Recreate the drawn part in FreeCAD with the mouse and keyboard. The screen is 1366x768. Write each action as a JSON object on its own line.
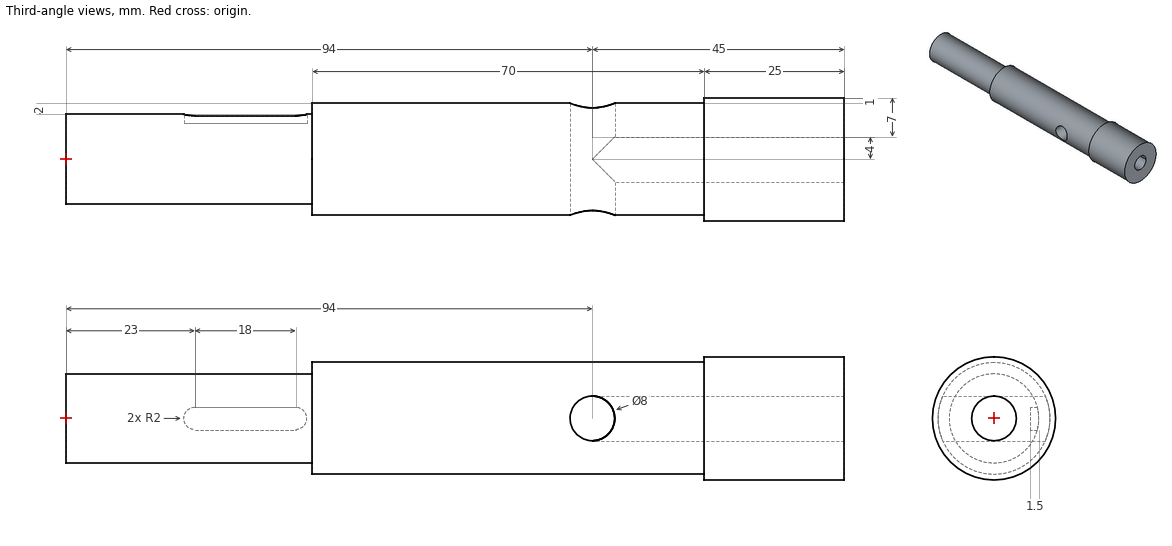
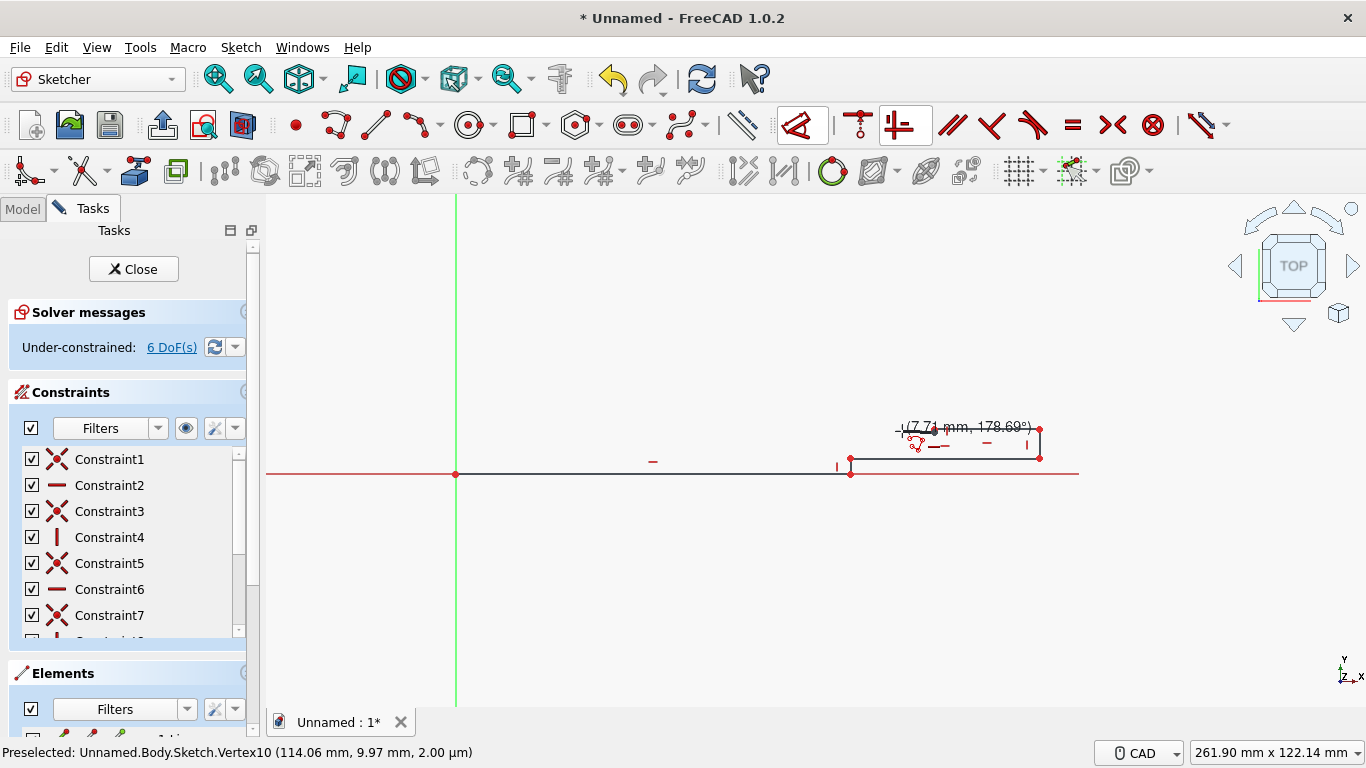
{"action": "left_click", "coordinate": [641, 432]}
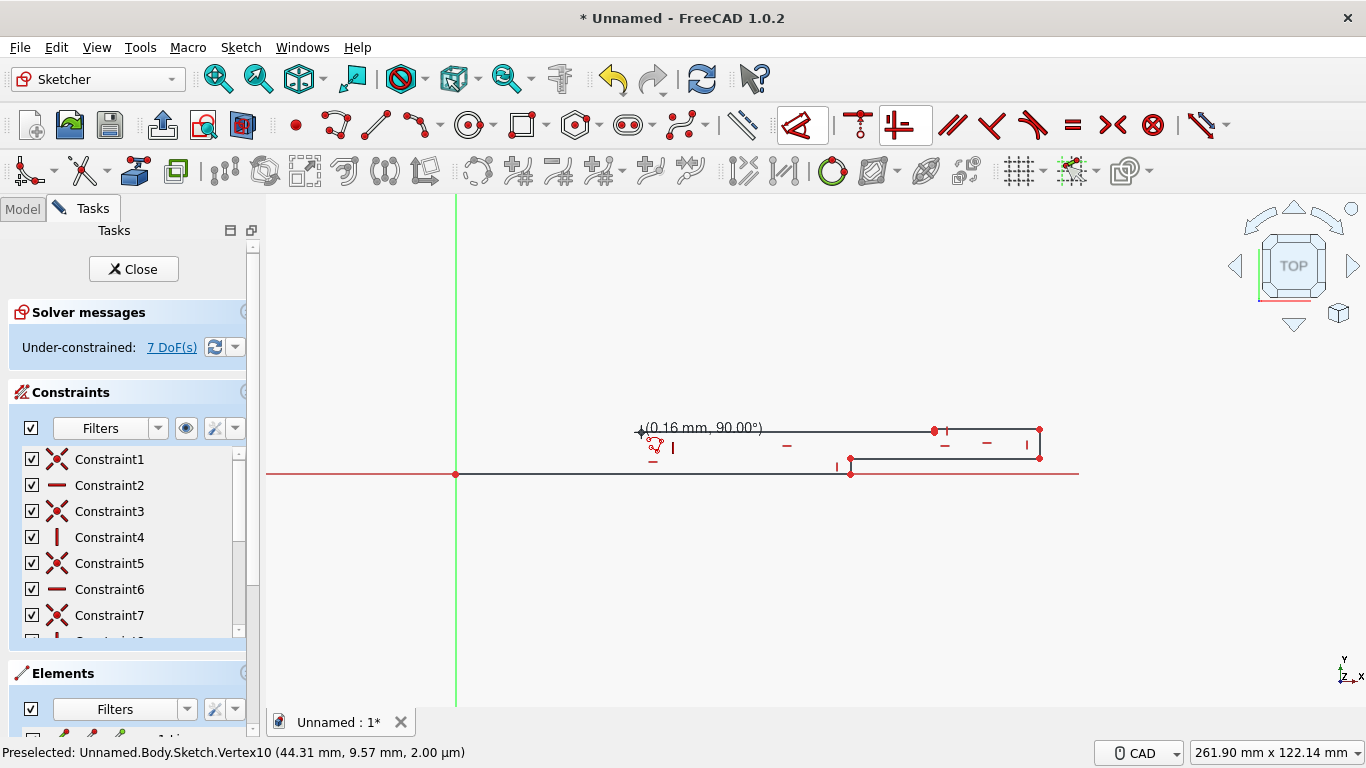
{"action": "scroll", "coordinate": [641, 441], "scroll_direction": "up", "scroll_amount": 4}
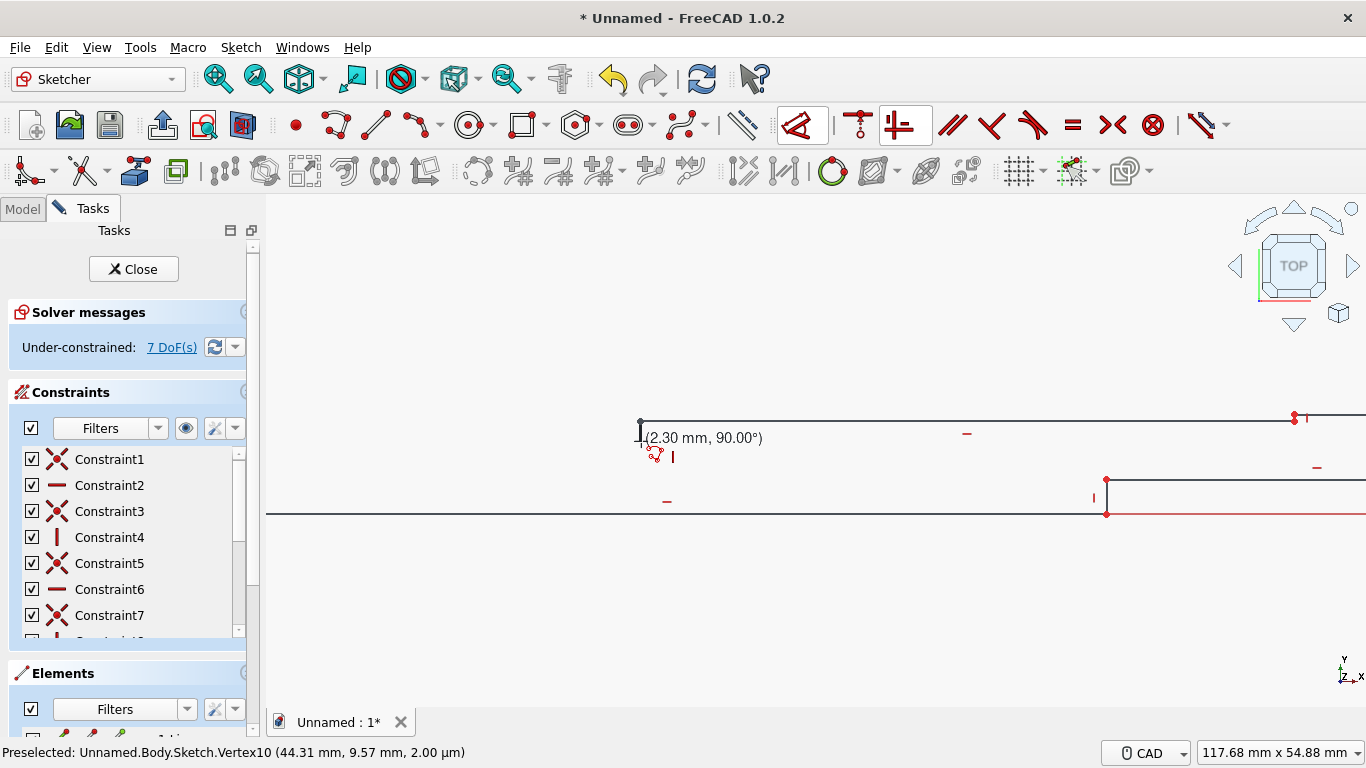
{"action": "left_click", "coordinate": [641, 440]}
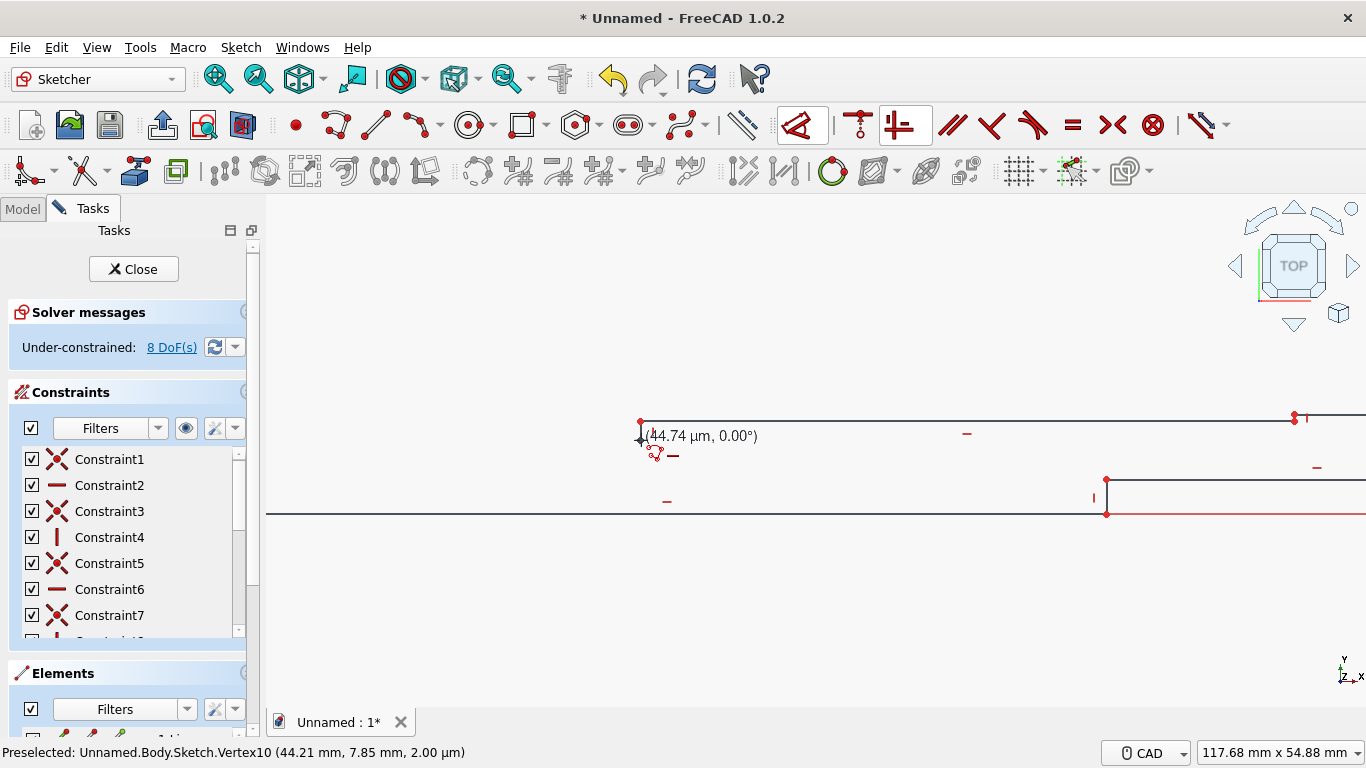
{"action": "scroll", "coordinate": [641, 440], "scroll_direction": "down", "scroll_amount": 4}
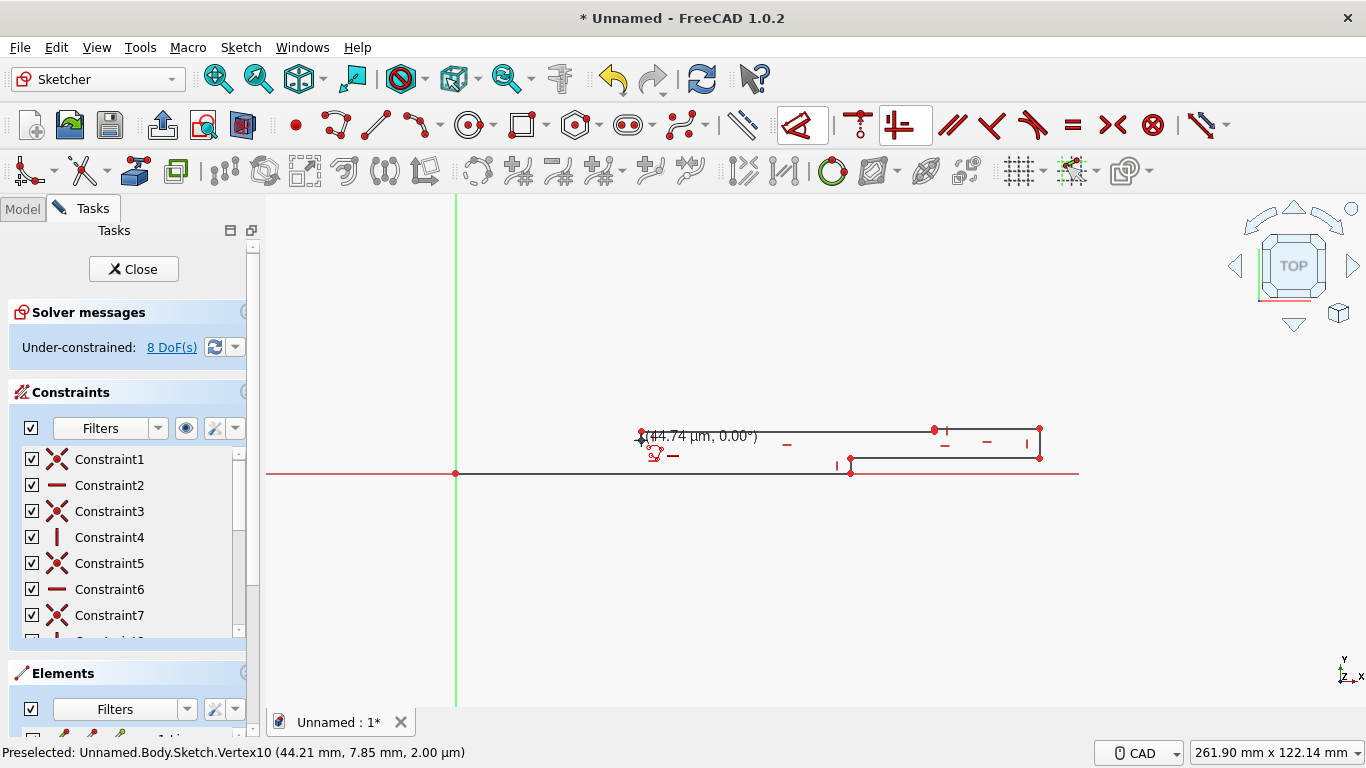
{"action": "left_click", "coordinate": [465, 440]}
{"action": "left_click", "coordinate": [456, 474]}
{"action": "key", "text": "Escape"}
{"action": "key", "text": "Escape"}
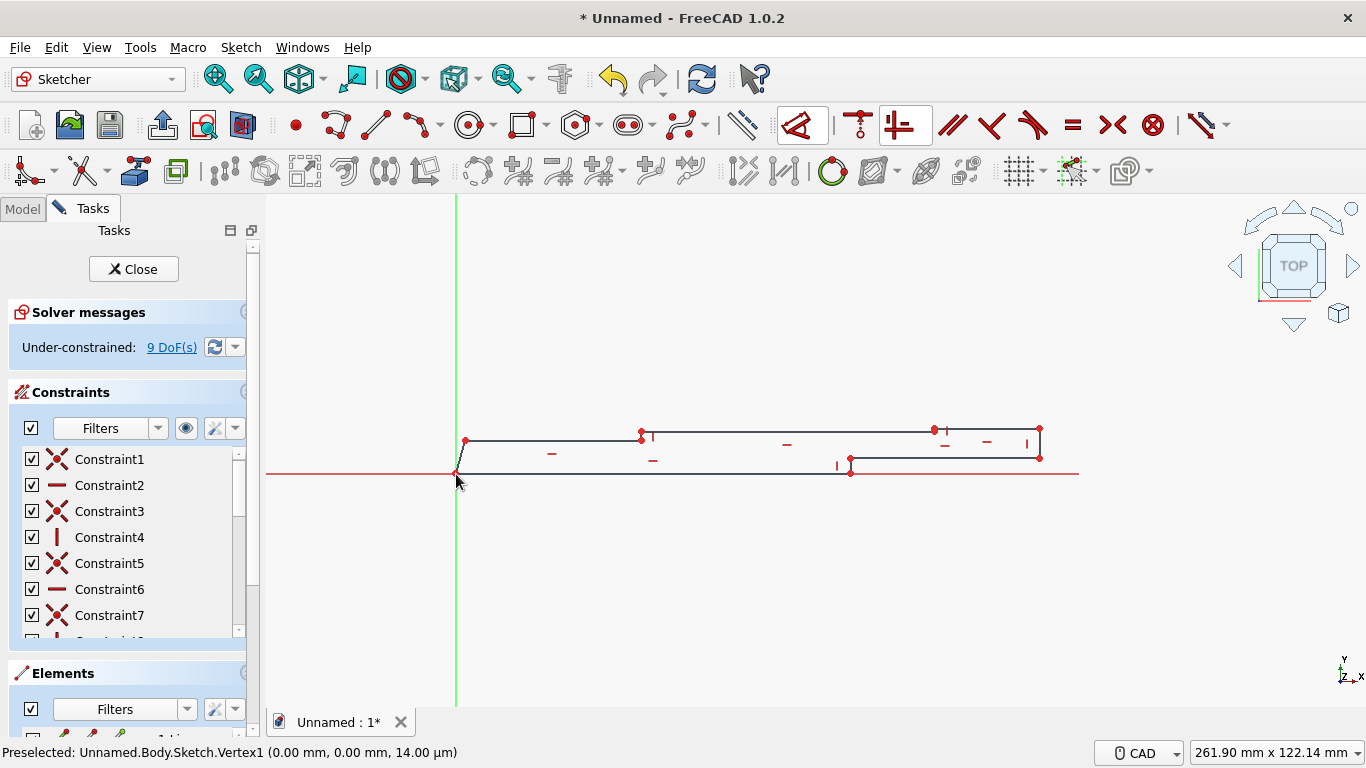
{"action": "scroll", "coordinate": [459, 464], "scroll_direction": "up", "scroll_amount": 2}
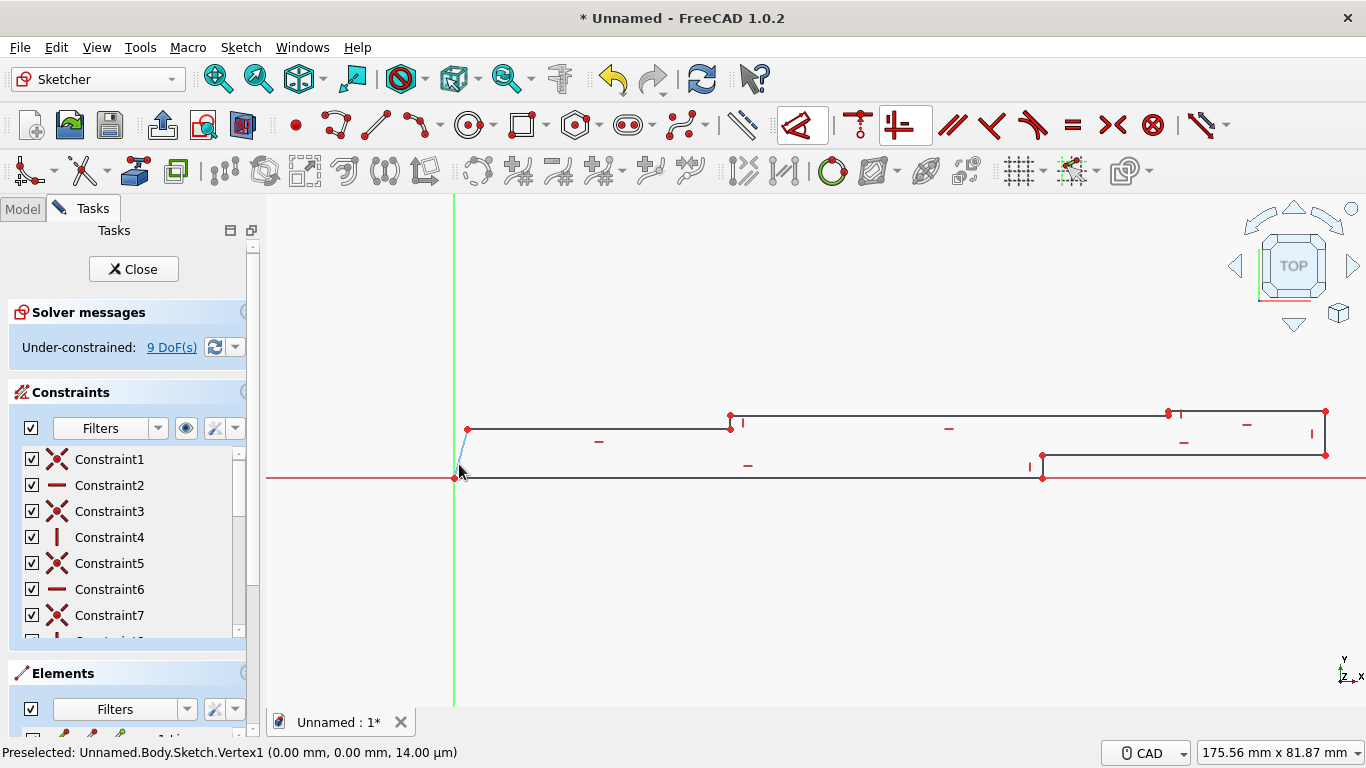
{"action": "left_click", "coordinate": [458, 463]}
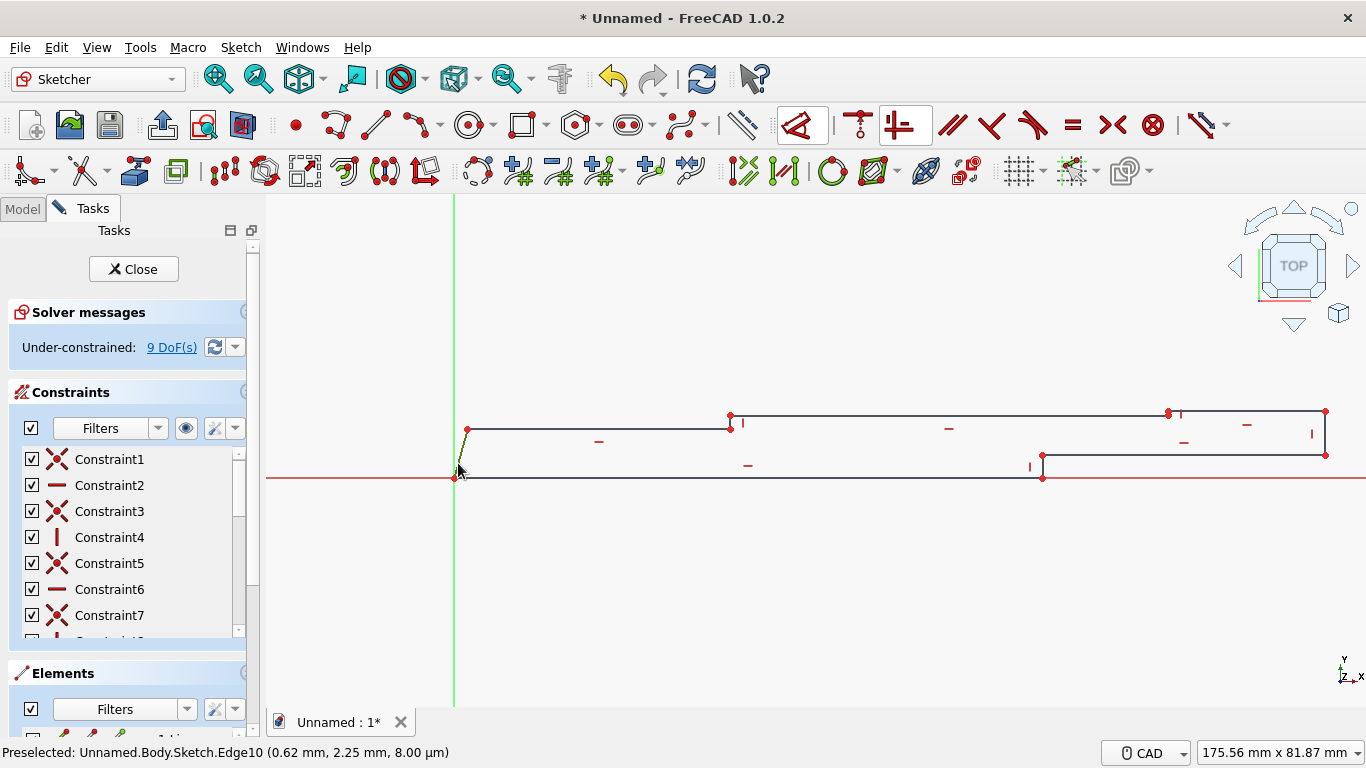
{"action": "left_click", "coordinate": [926, 126]}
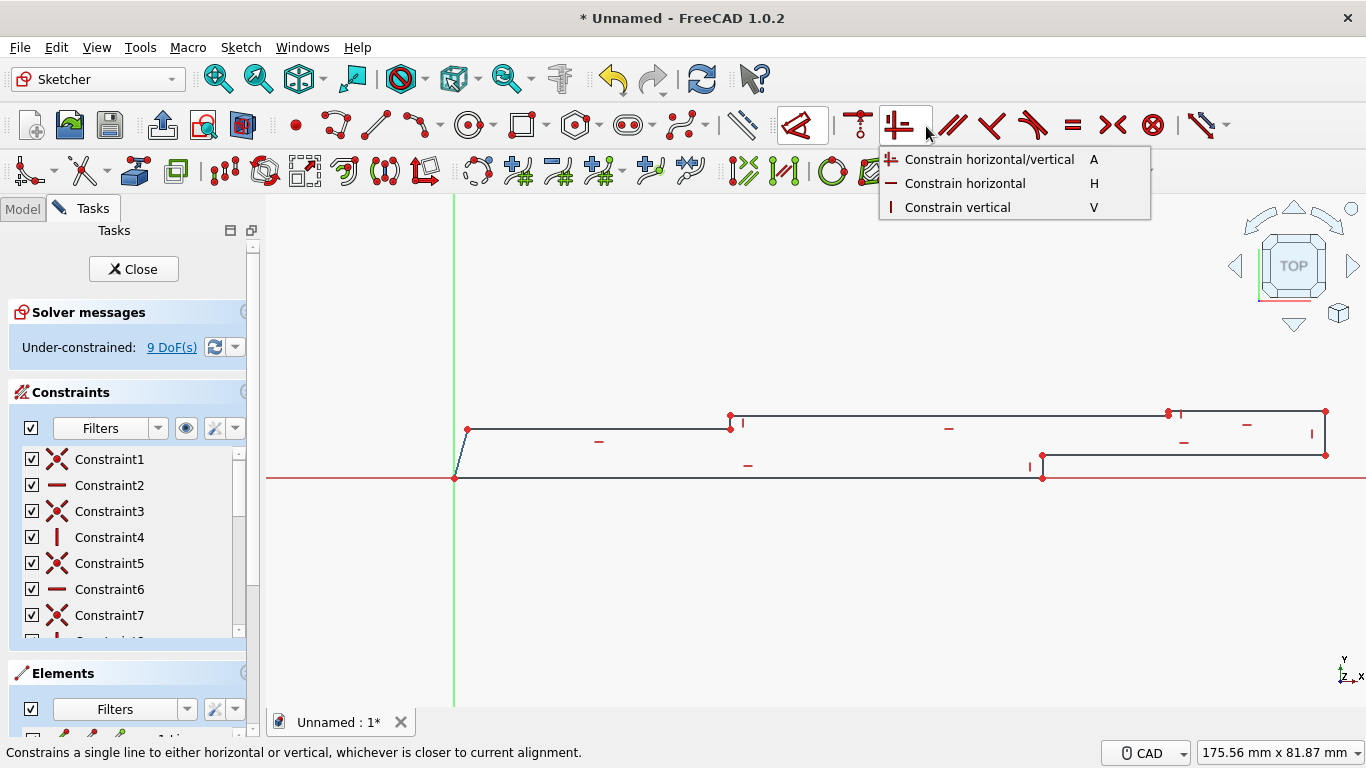
{"action": "left_click", "coordinate": [1015, 207]}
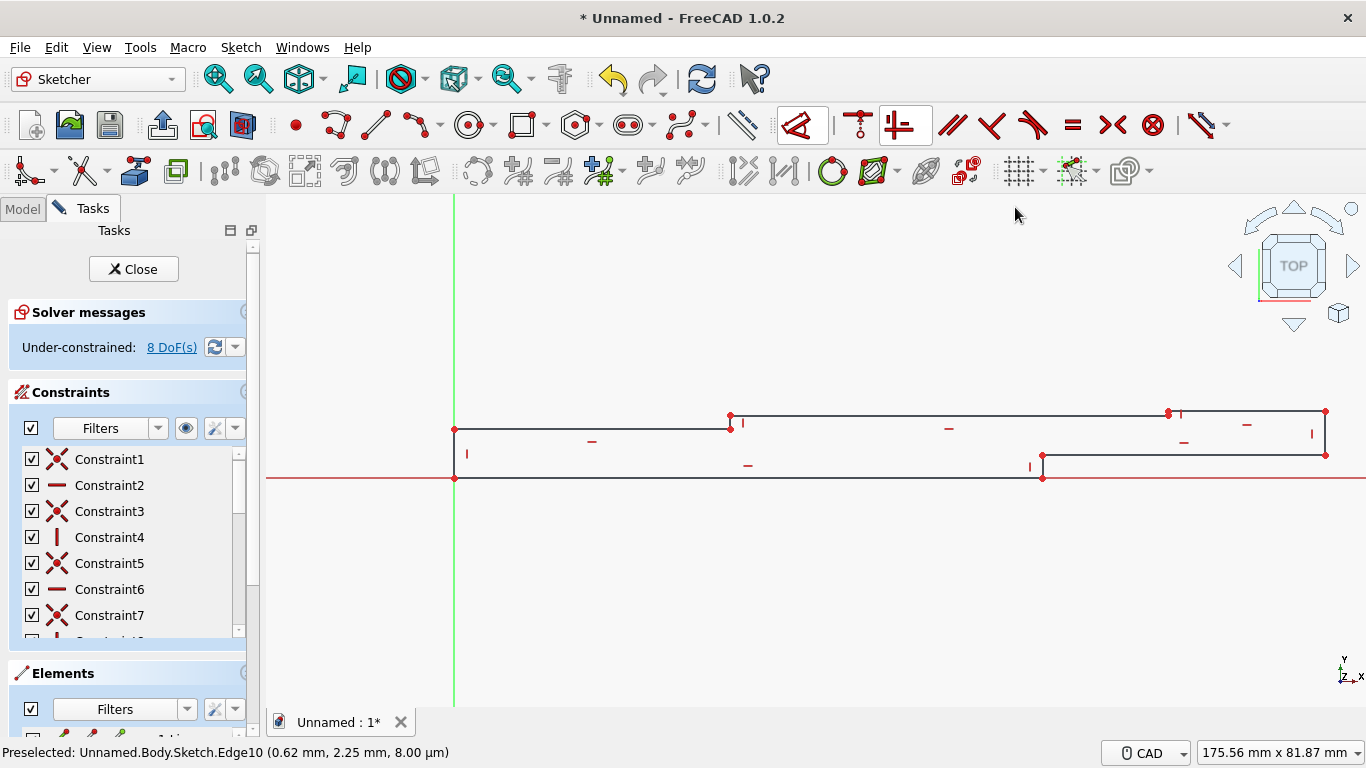
{"action": "left_click", "coordinate": [796, 126]}